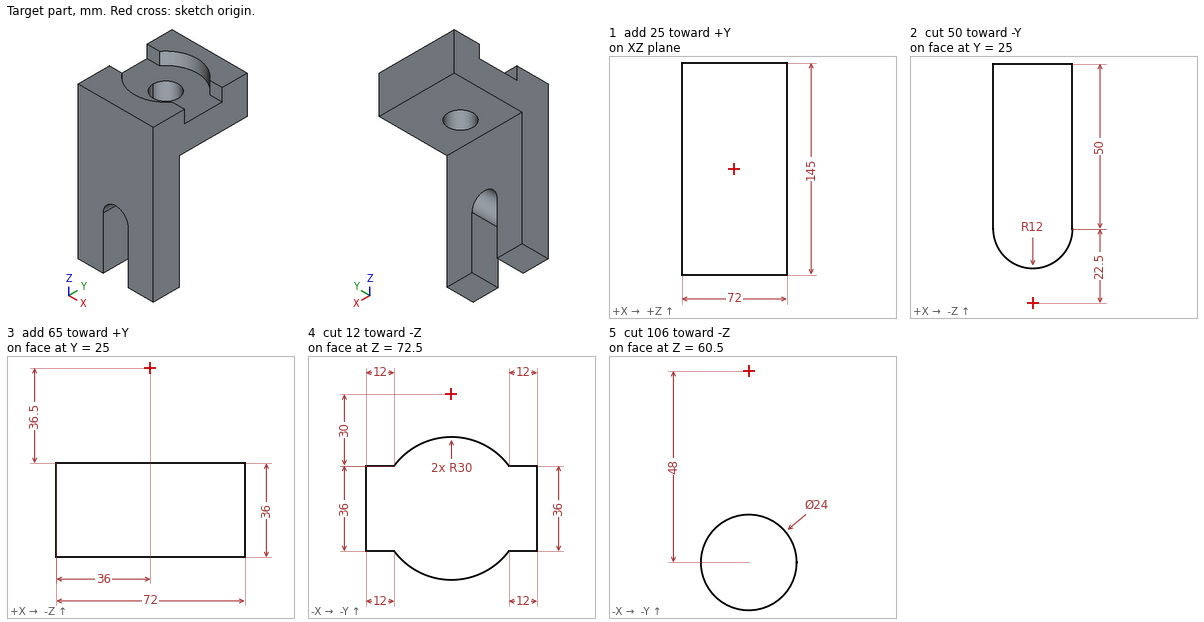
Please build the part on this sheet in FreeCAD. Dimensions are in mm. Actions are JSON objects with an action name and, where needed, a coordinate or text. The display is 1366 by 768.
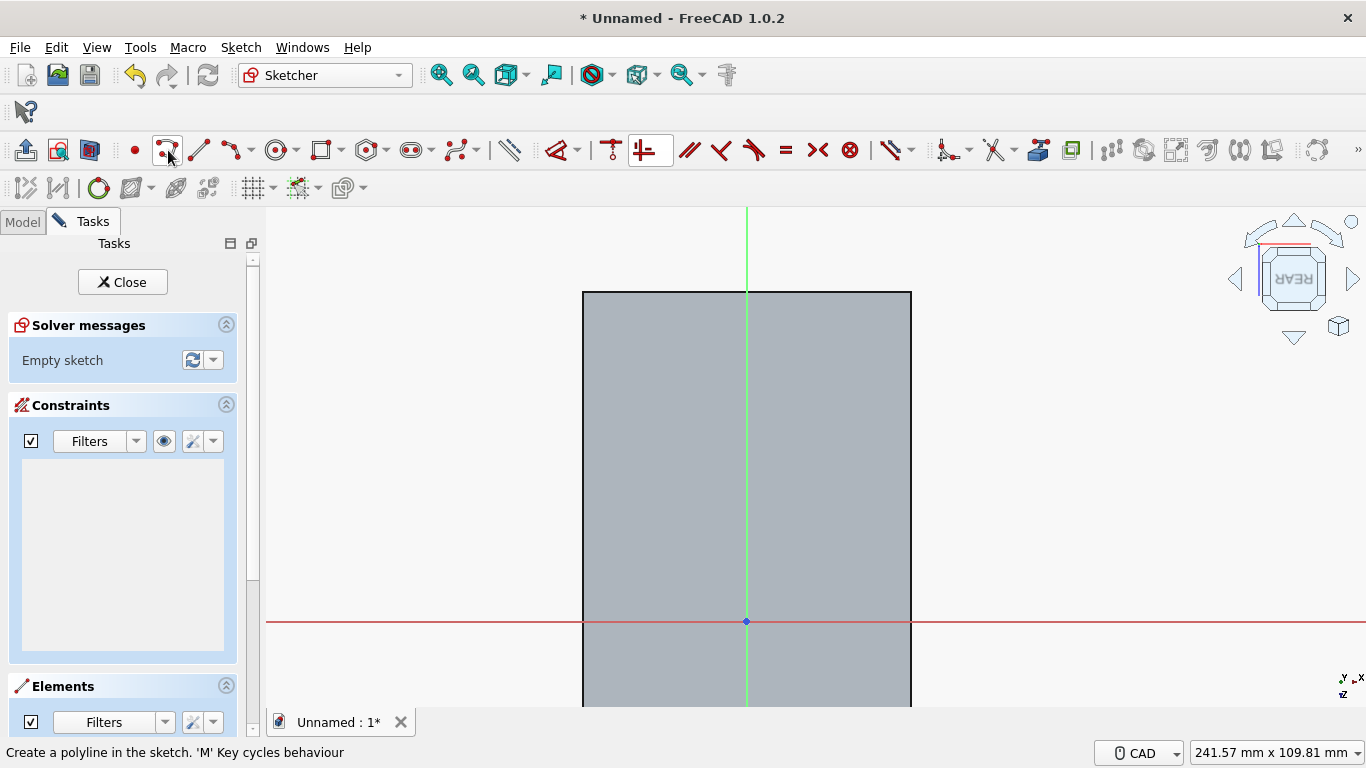
{"action": "left_click", "coordinate": [801, 519]}
{"action": "left_click", "coordinate": [801, 292]}
{"action": "left_click", "coordinate": [692, 292]}
{"action": "left_click", "coordinate": [692, 519]}
{"action": "right_click", "coordinate": [692, 519]}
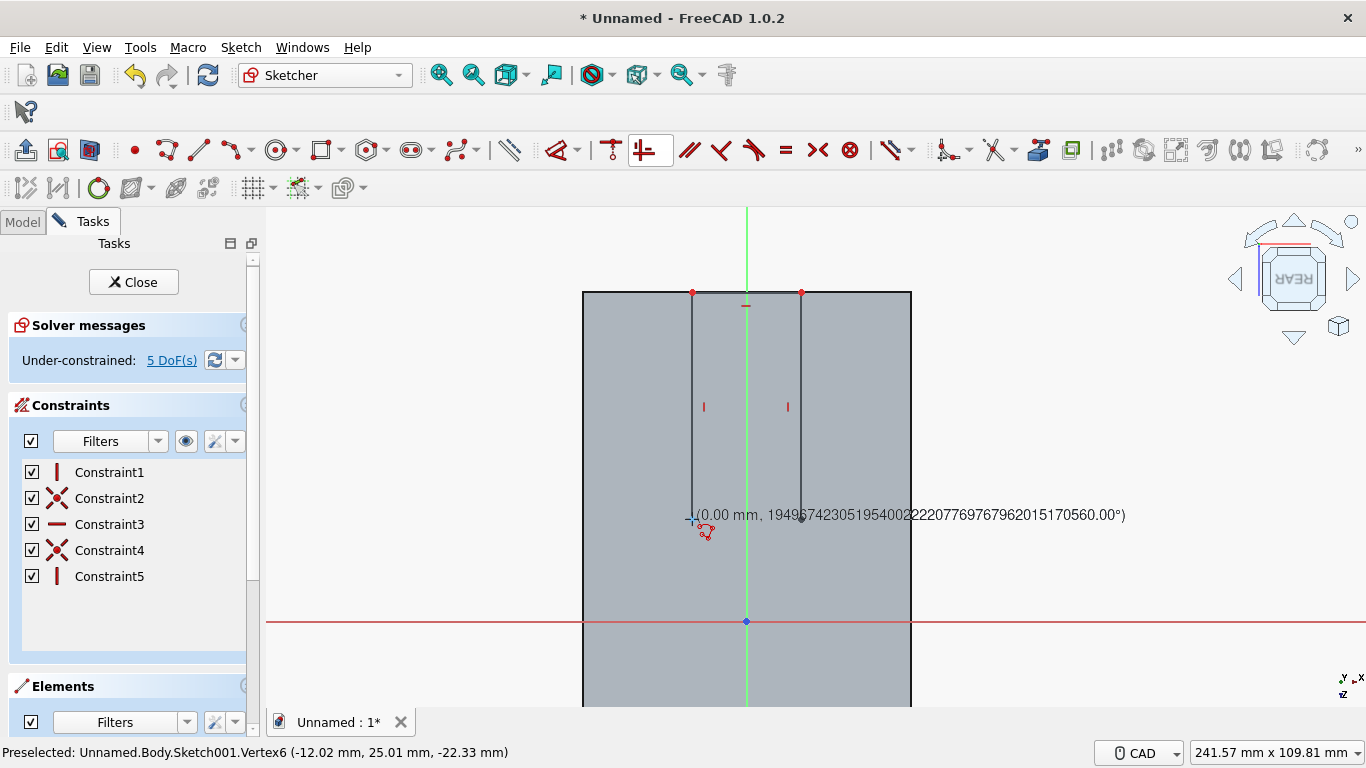
{"action": "left_click", "coordinate": [232, 150]}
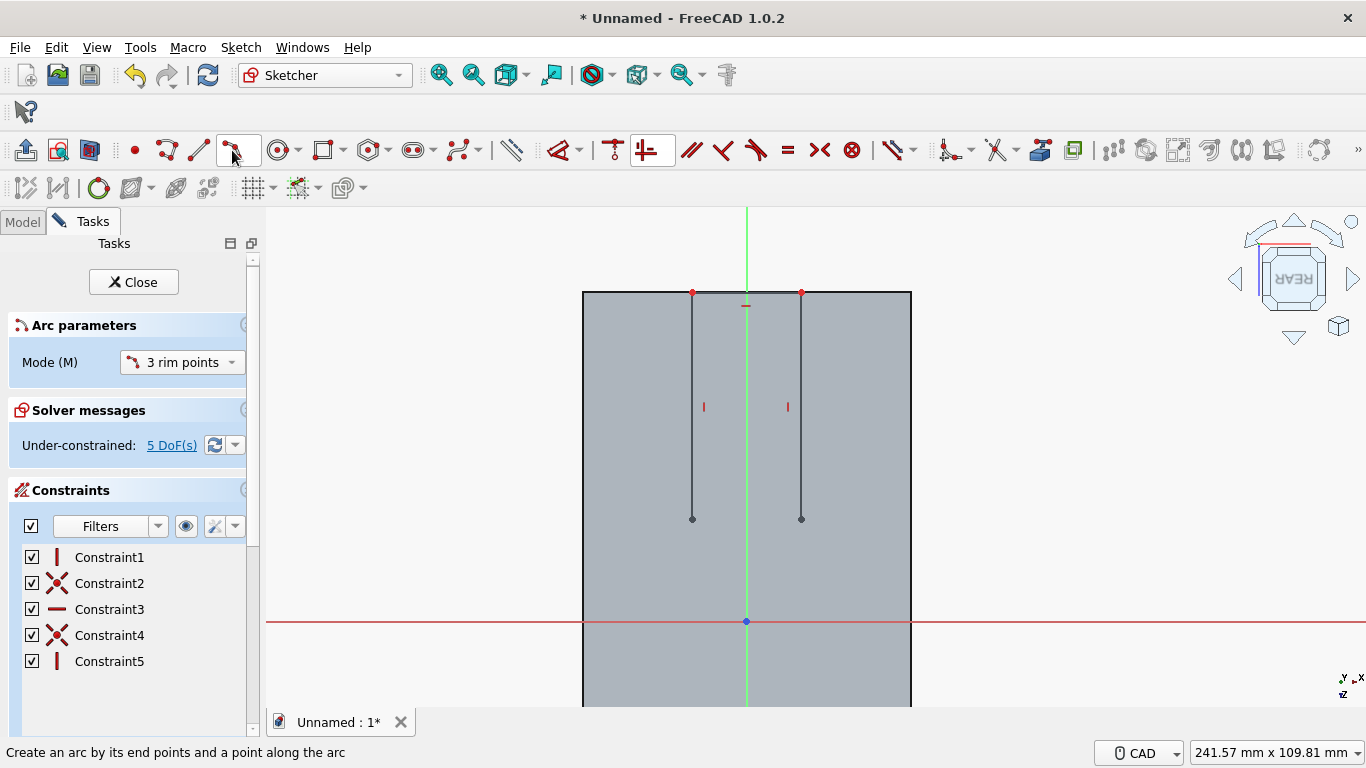
{"action": "left_click", "coordinate": [692, 520]}
{"action": "left_click", "coordinate": [801, 520]}
{"action": "left_click", "coordinate": [730, 571]}
{"action": "key", "text": "Escape"}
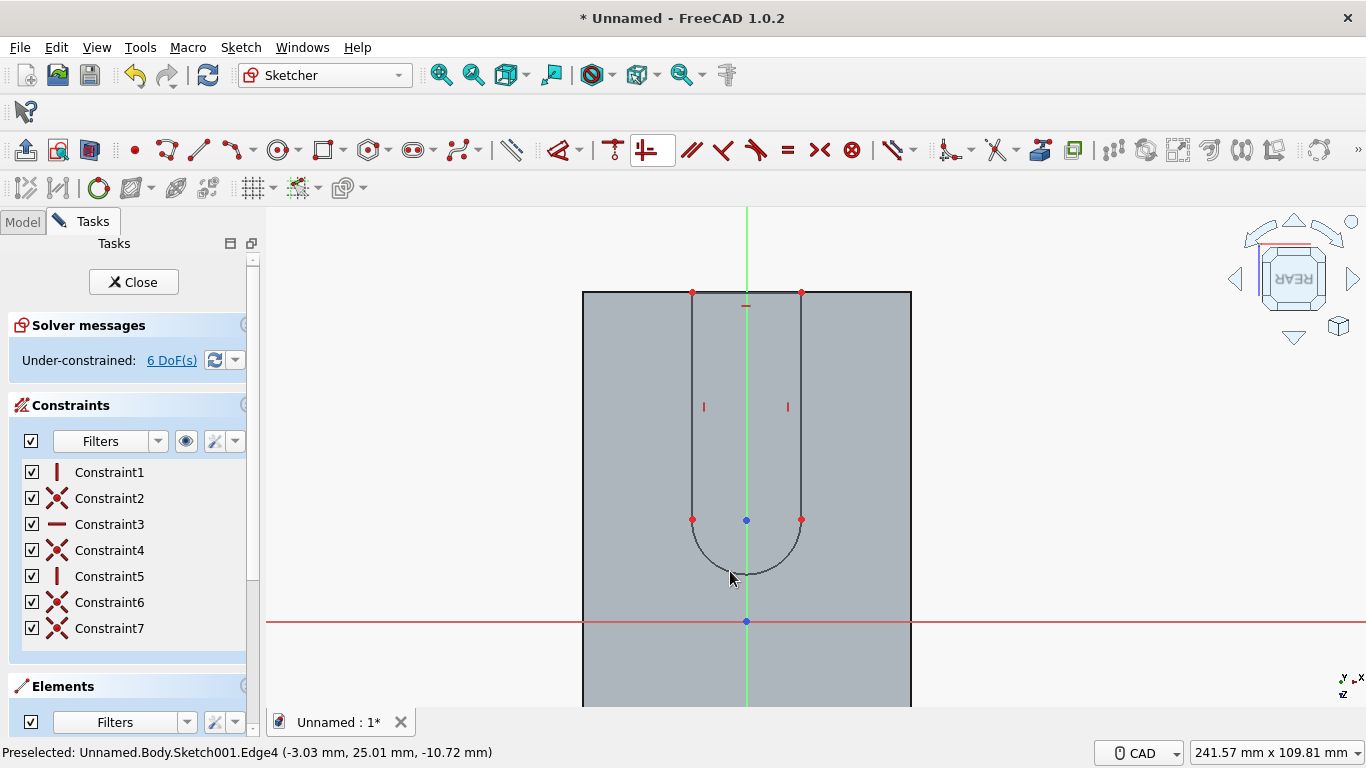
{"action": "left_click", "coordinate": [801, 452]}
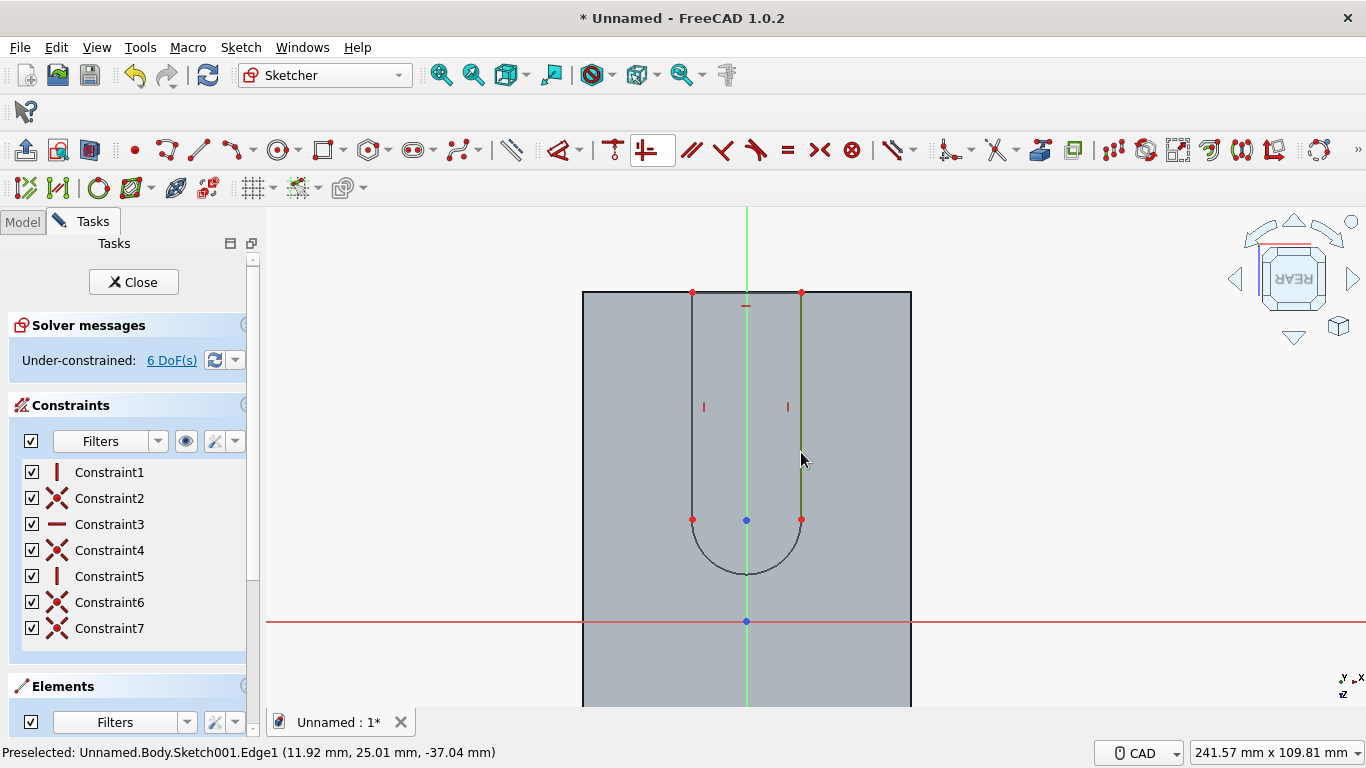
{"action": "left_click", "coordinate": [714, 564]}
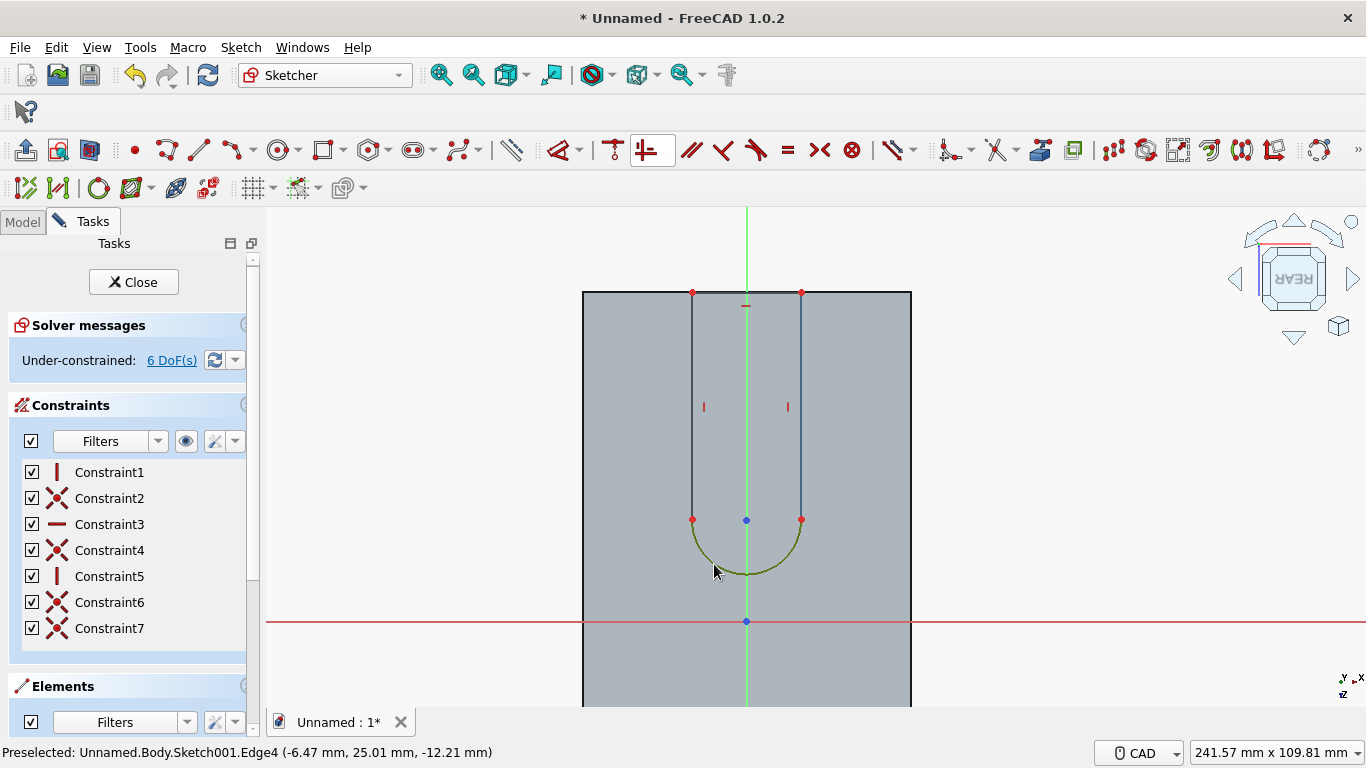
{"action": "left_click", "coordinate": [756, 150]}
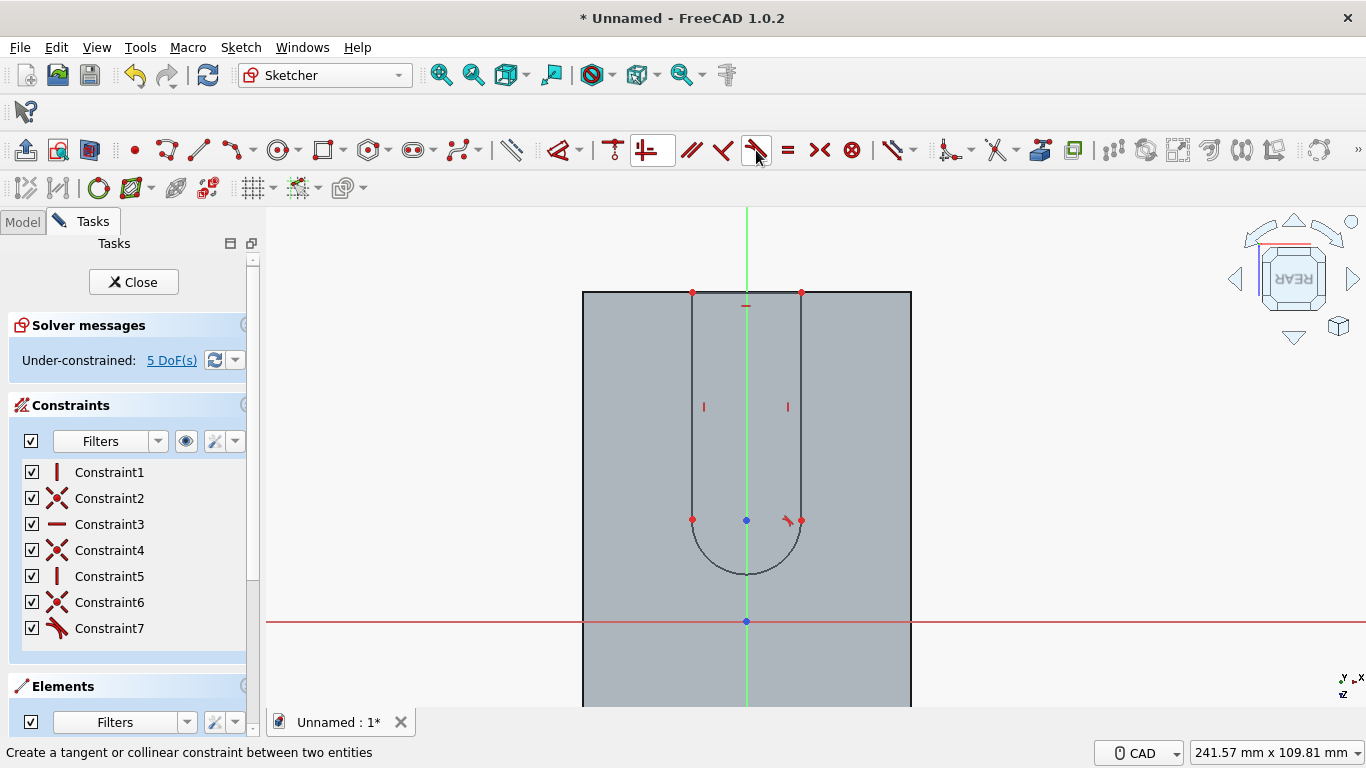
{"action": "left_click", "coordinate": [692, 361]}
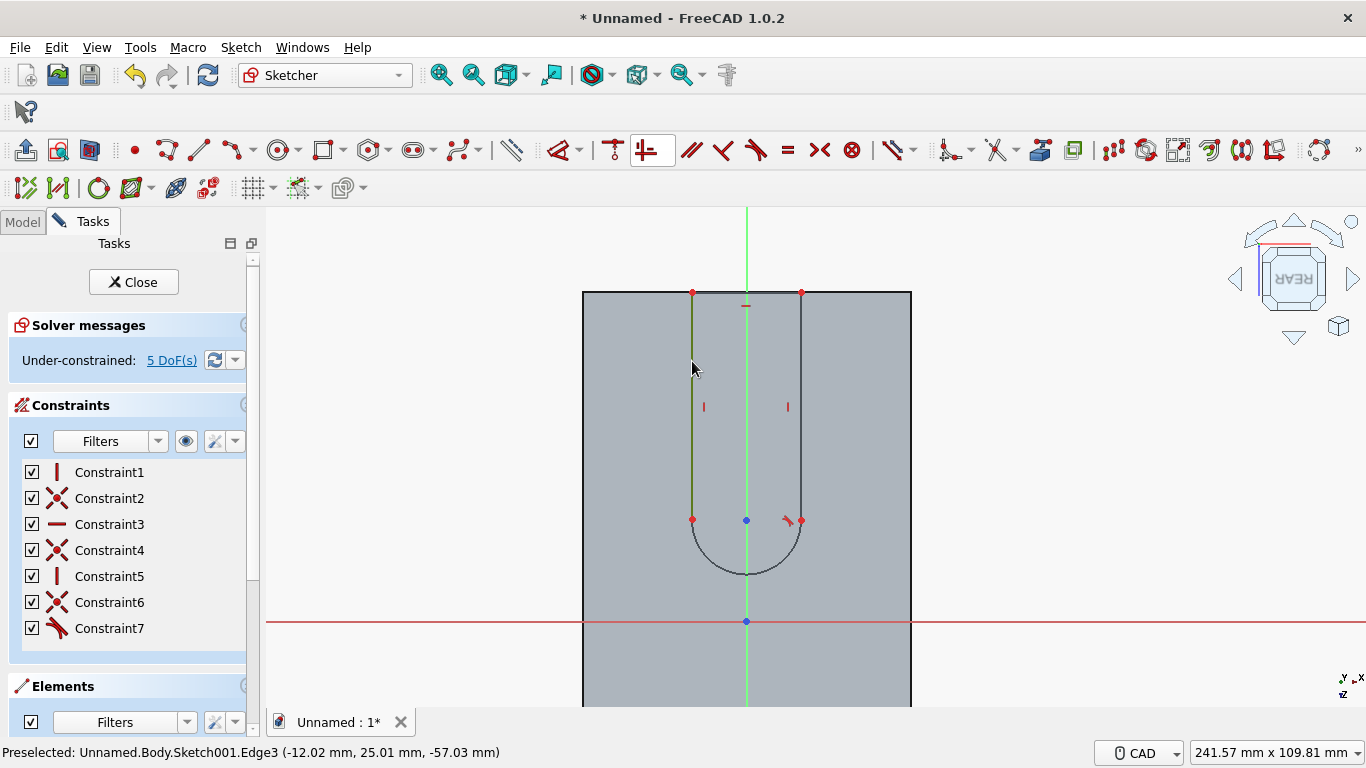
{"action": "left_click", "coordinate": [714, 564]}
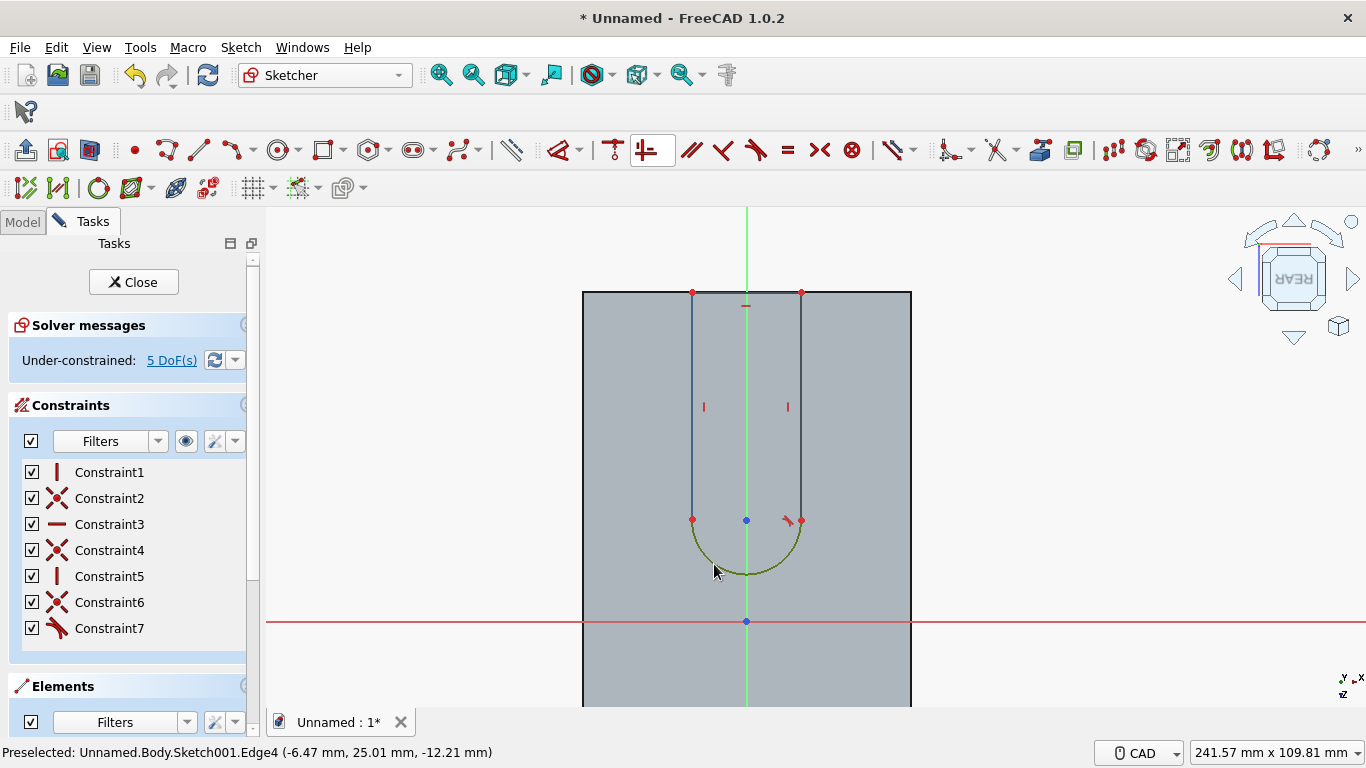
{"action": "left_click", "coordinate": [756, 150]}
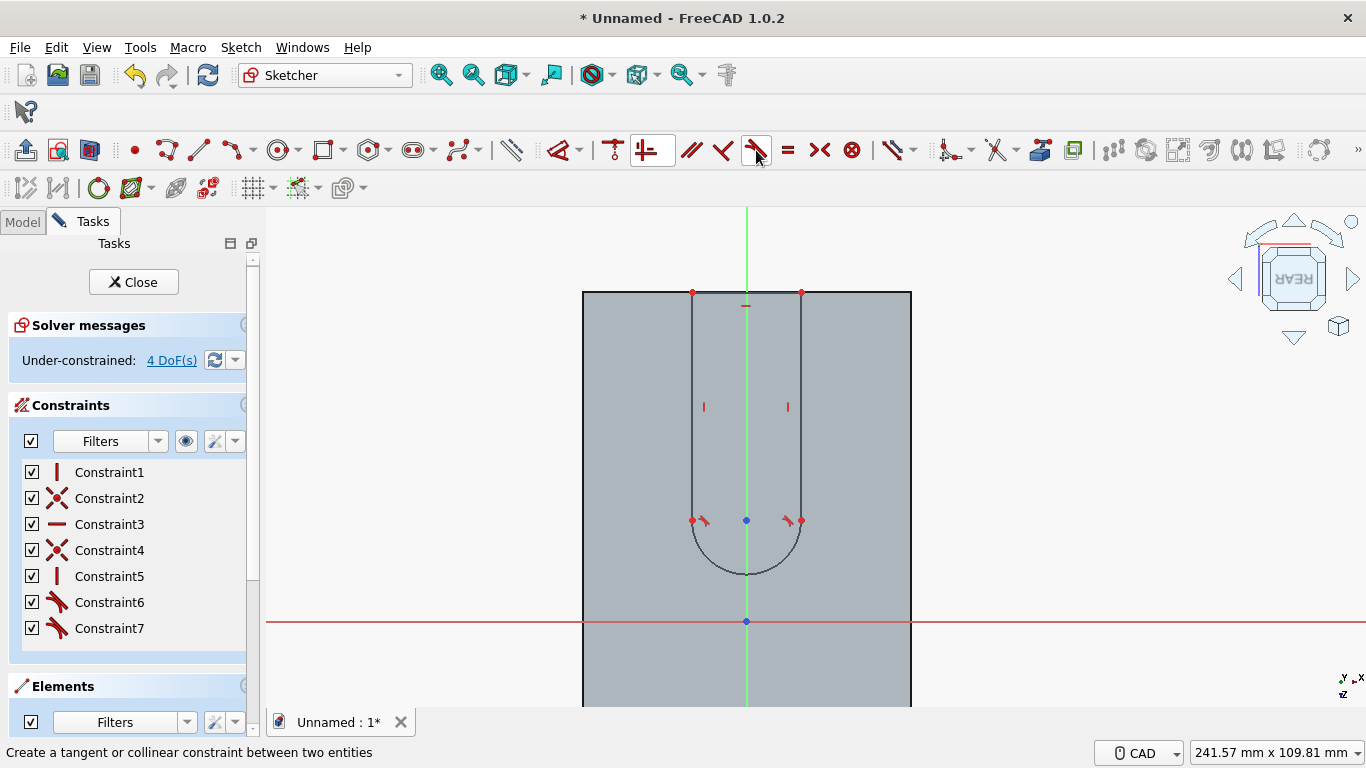
{"action": "left_click", "coordinate": [747, 520]}